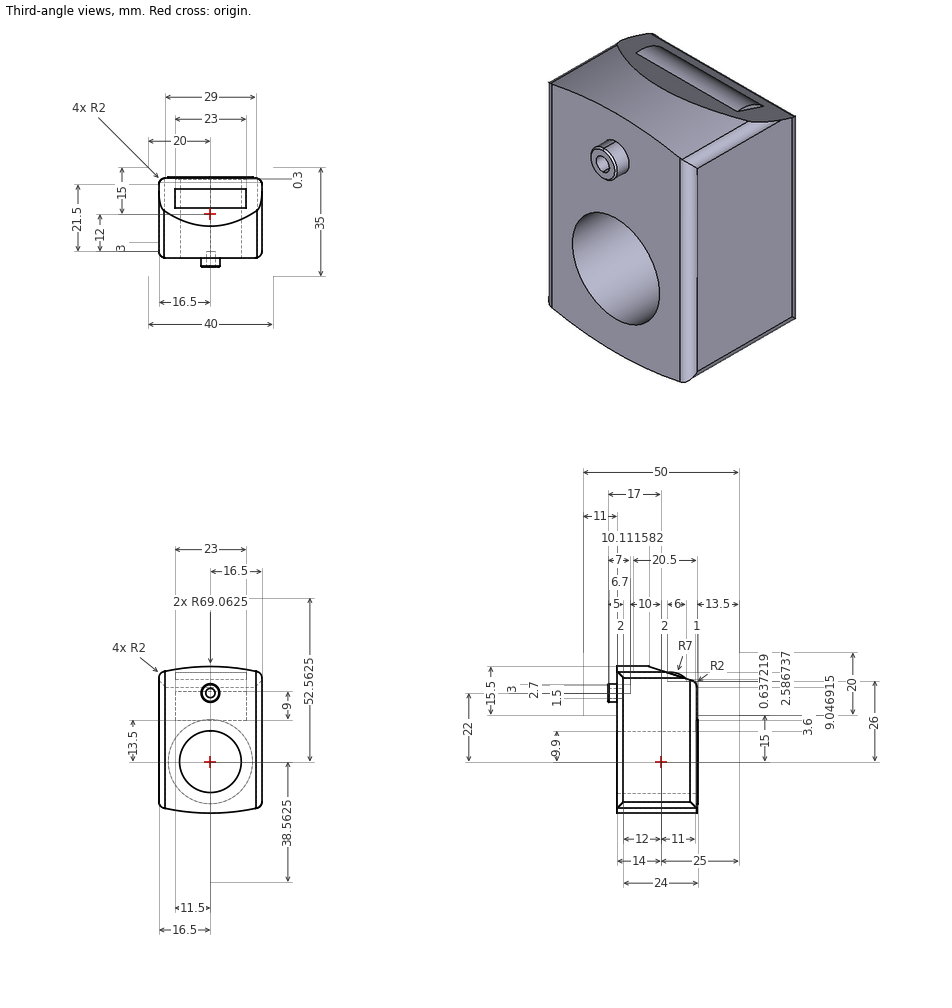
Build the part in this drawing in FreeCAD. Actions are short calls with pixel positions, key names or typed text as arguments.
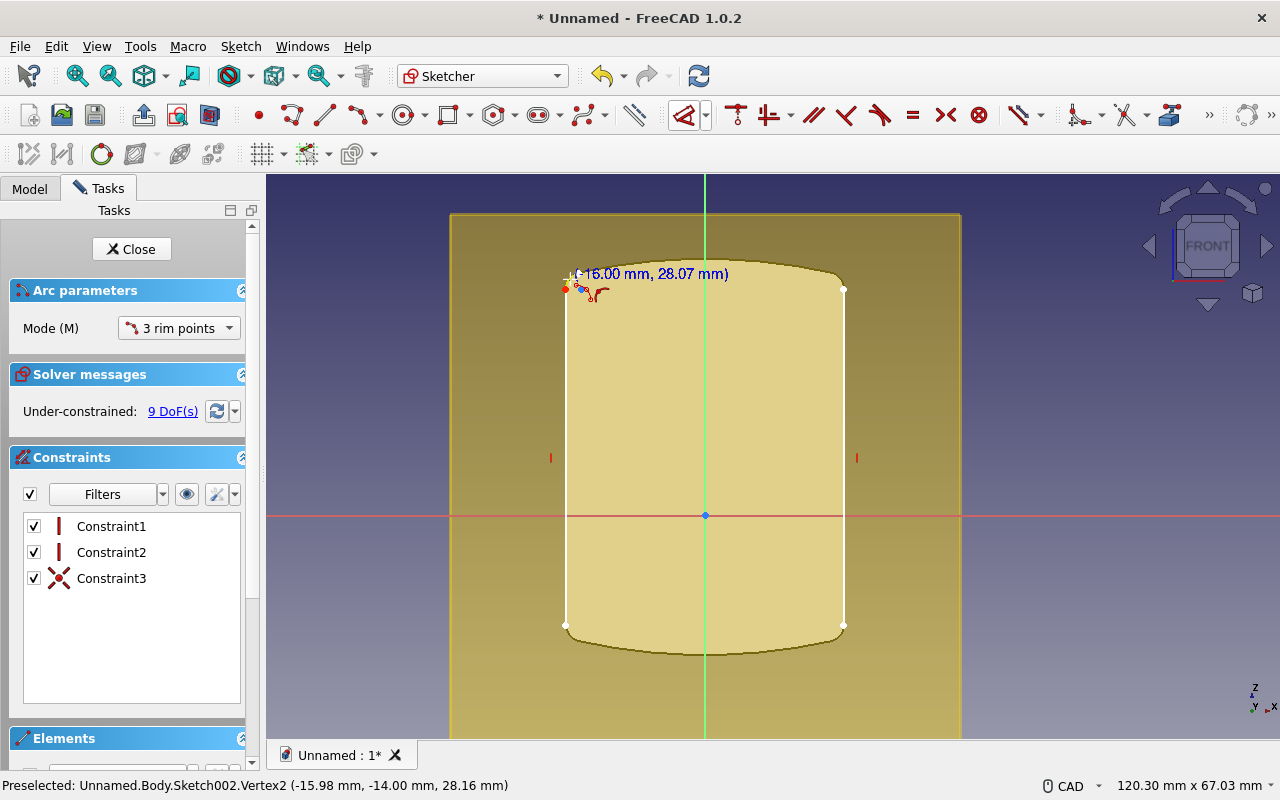
click(579, 274)
click(831, 273)
click(730, 259)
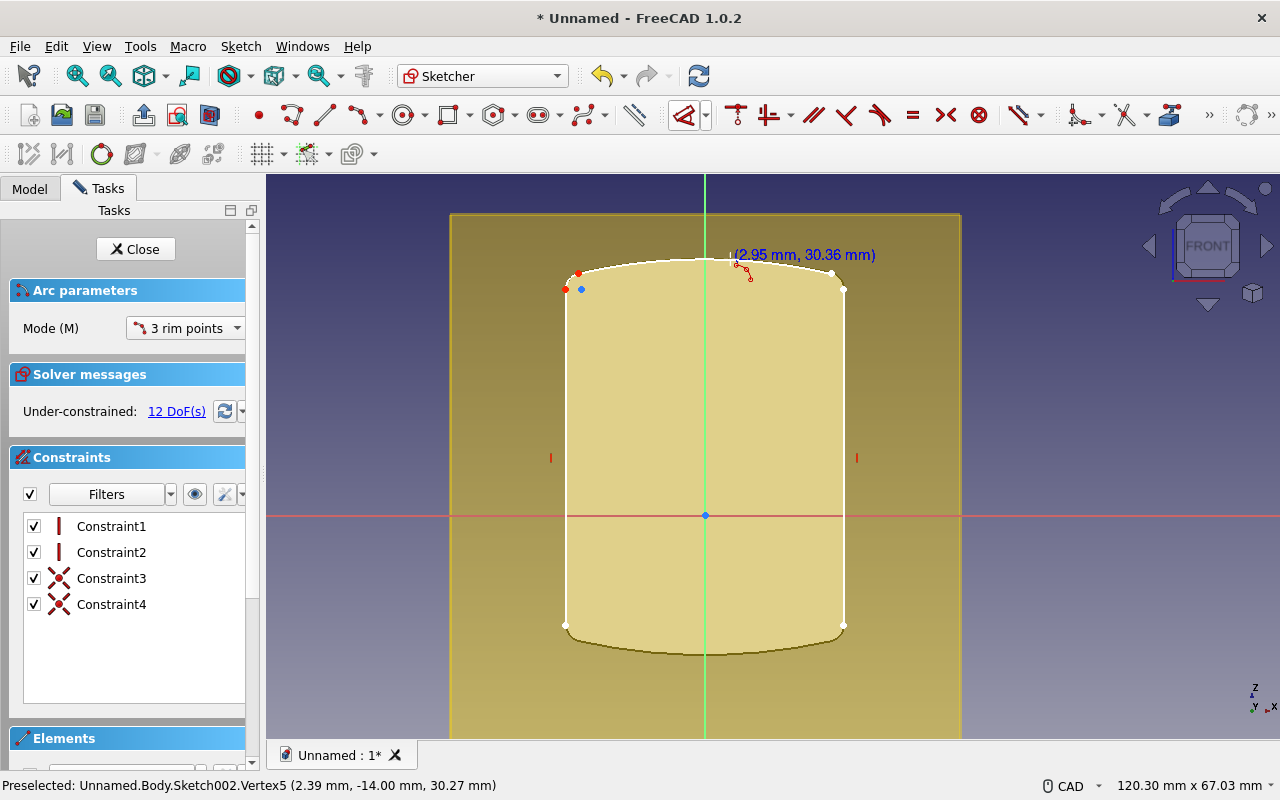
click(831, 274)
click(844, 290)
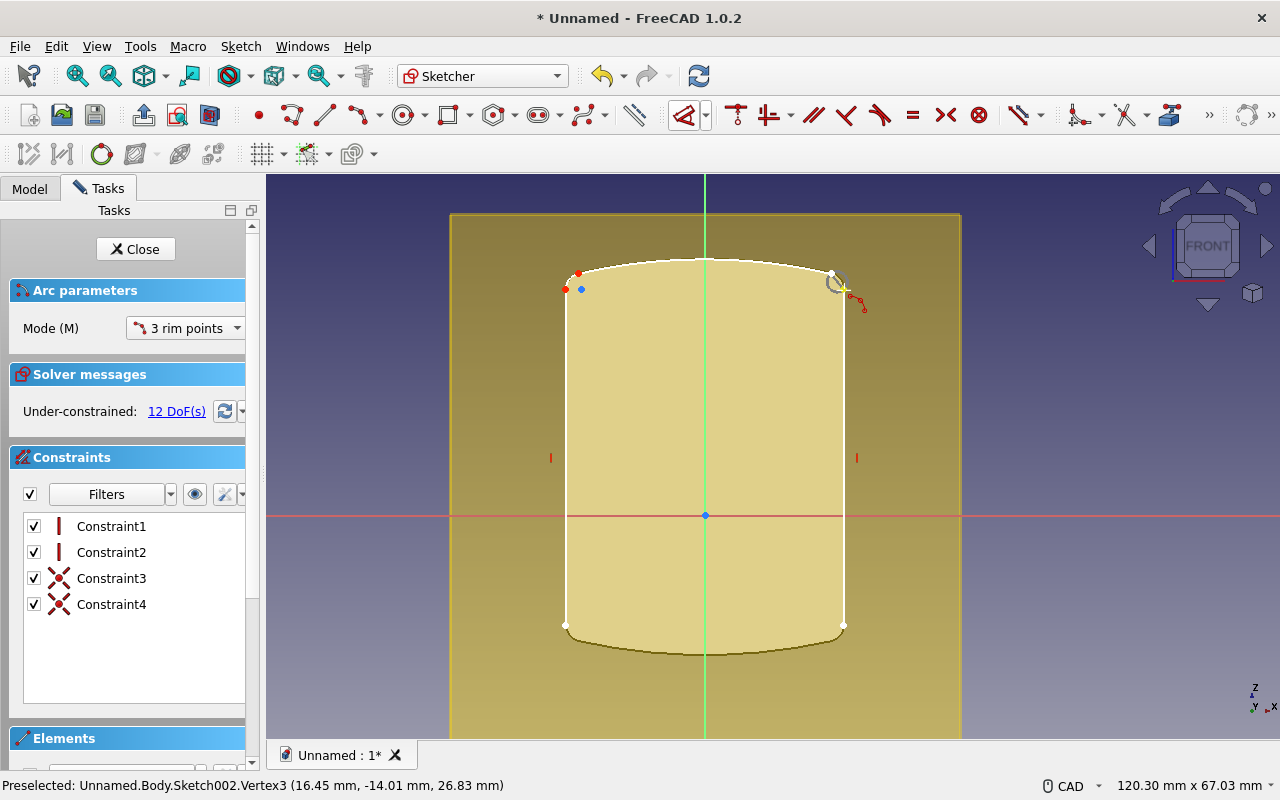
scroll(840, 279, up, 8)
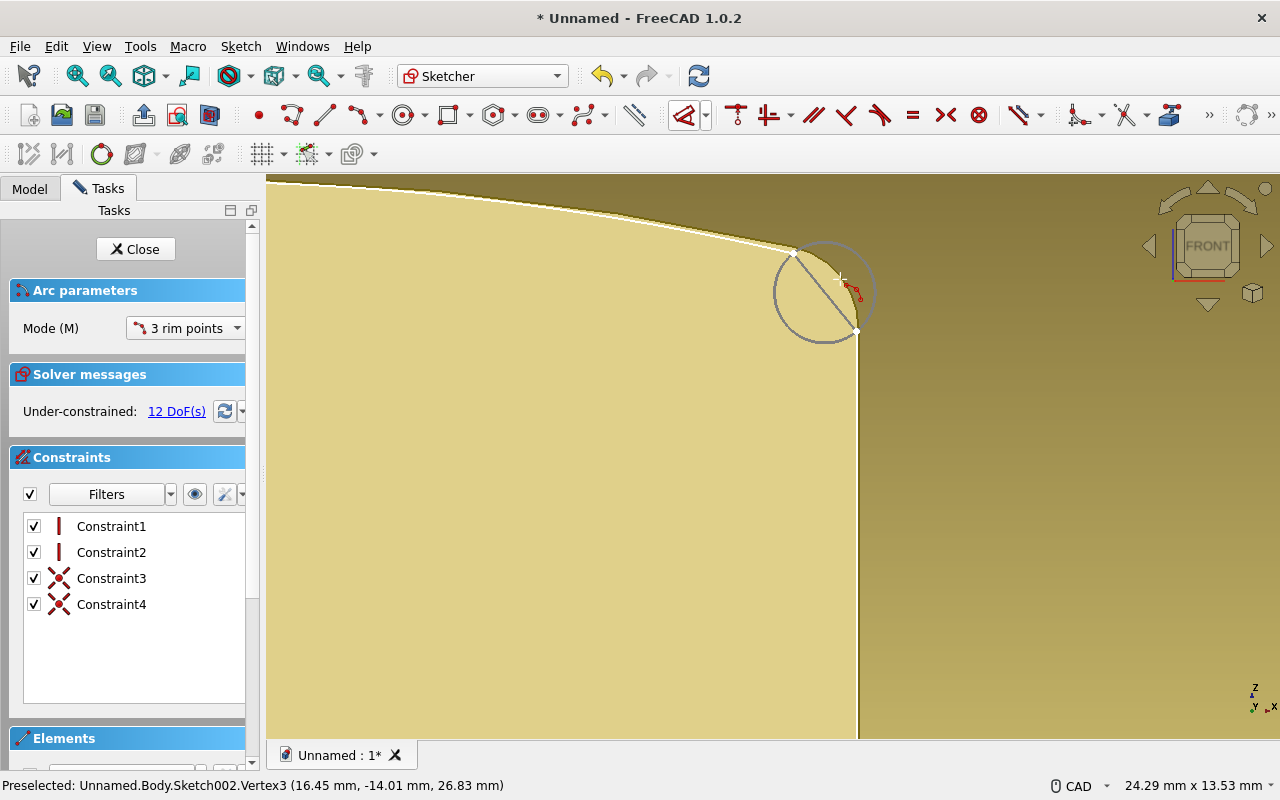
click(840, 276)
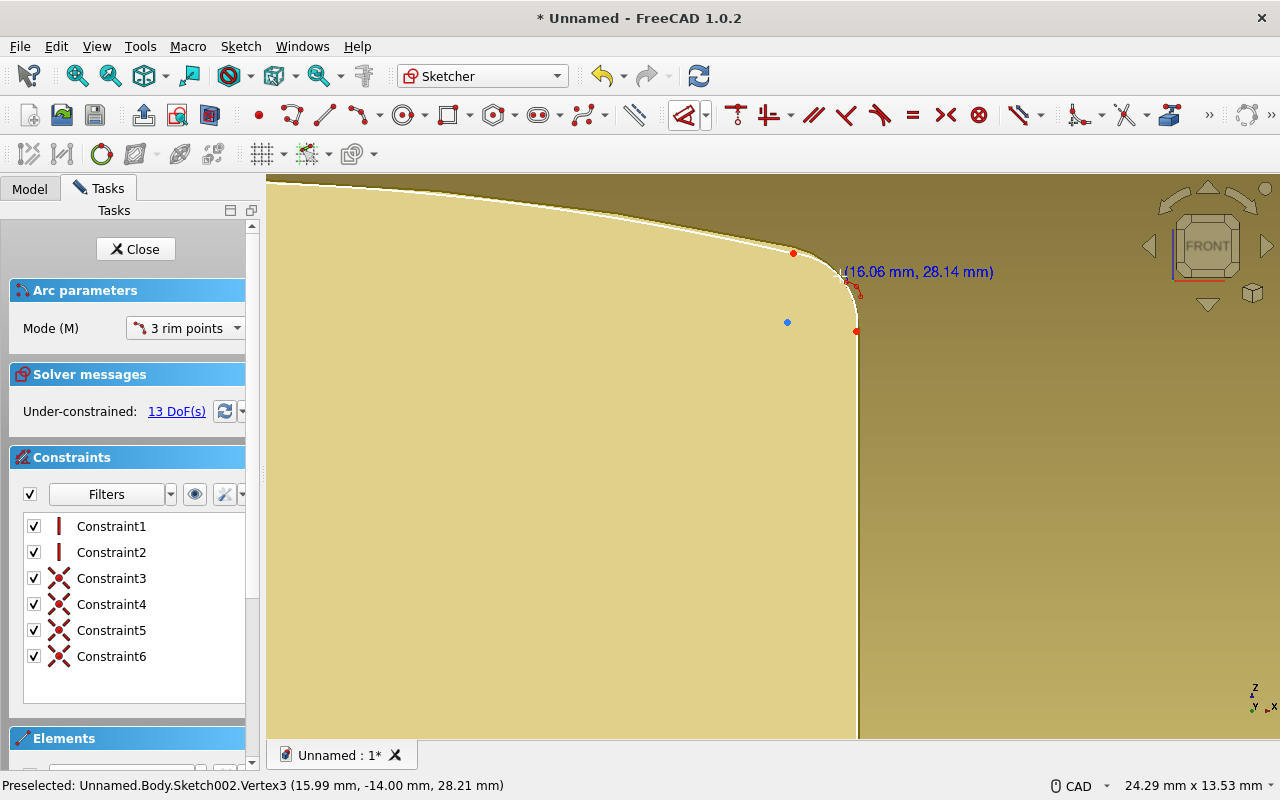
scroll(840, 279, down, 8)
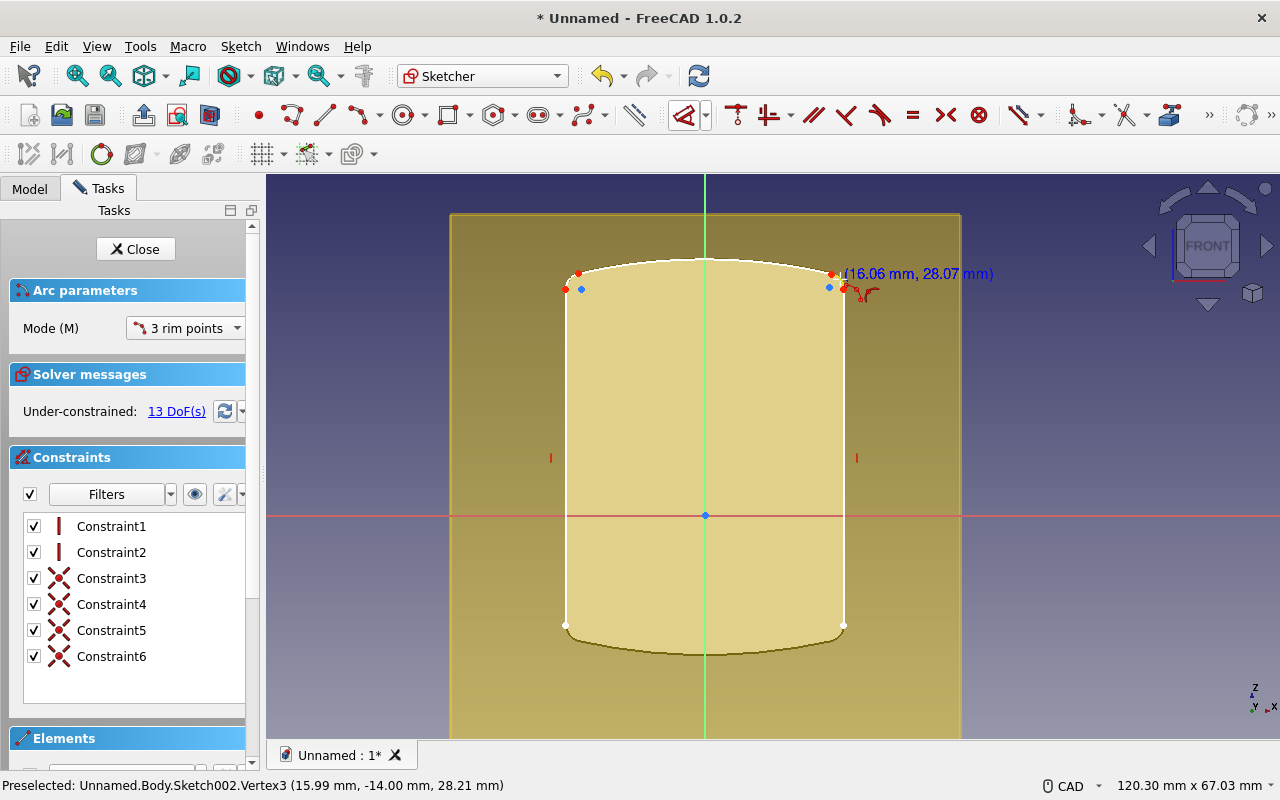
click(844, 626)
click(831, 641)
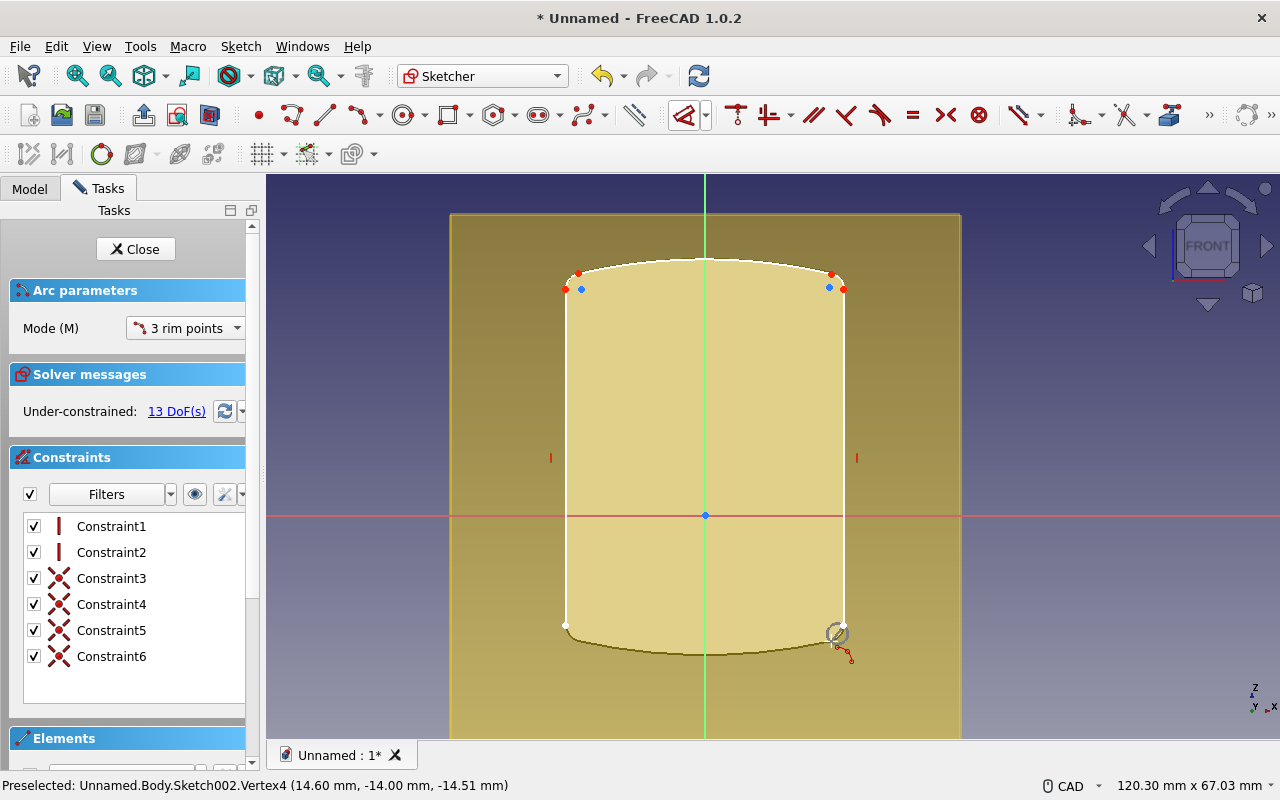
scroll(840, 635, up, 8)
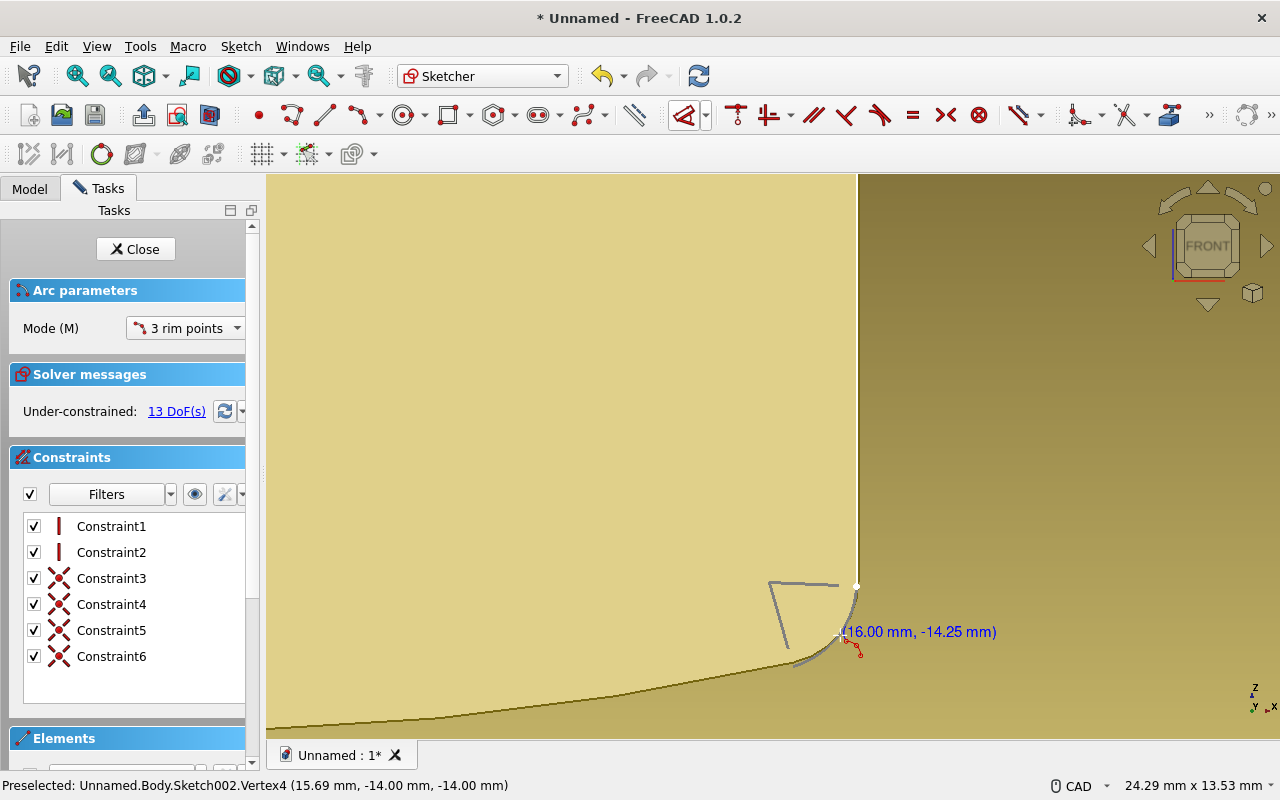
click(840, 633)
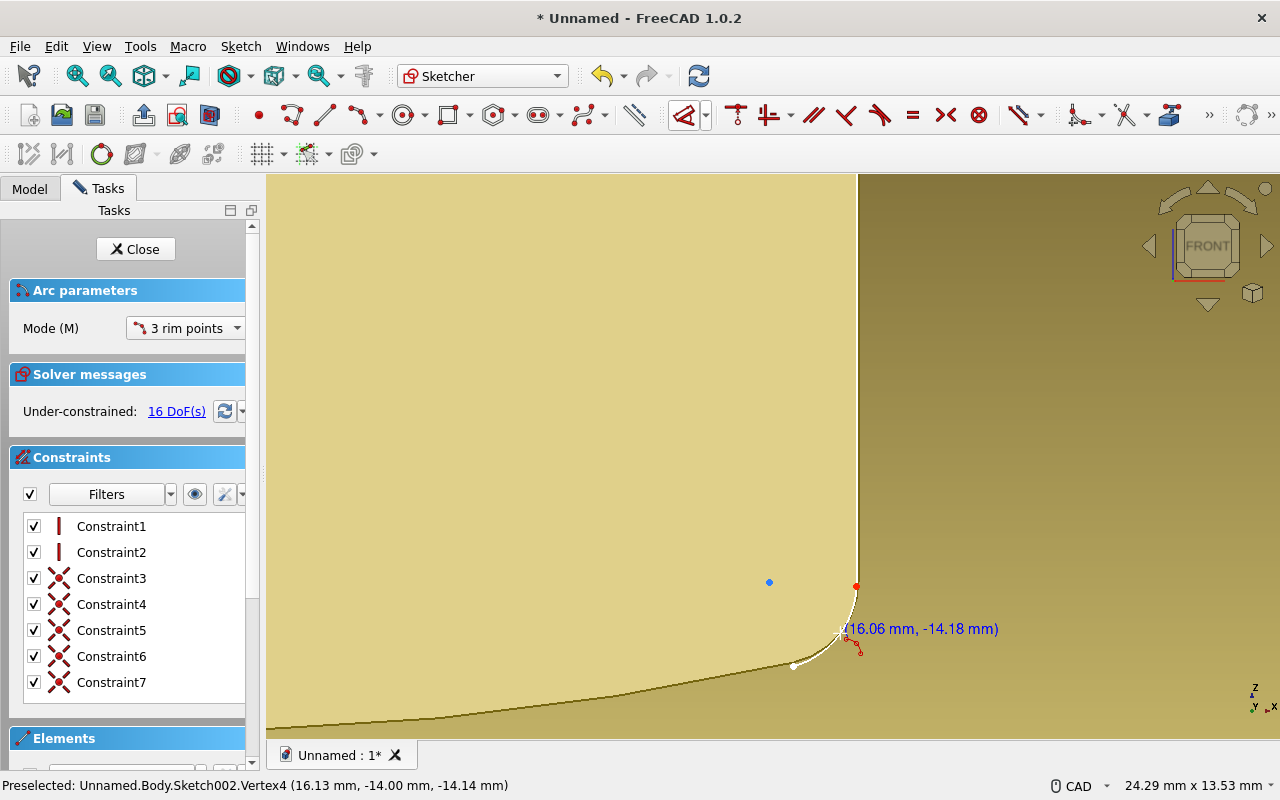
scroll(840, 635, down, 8)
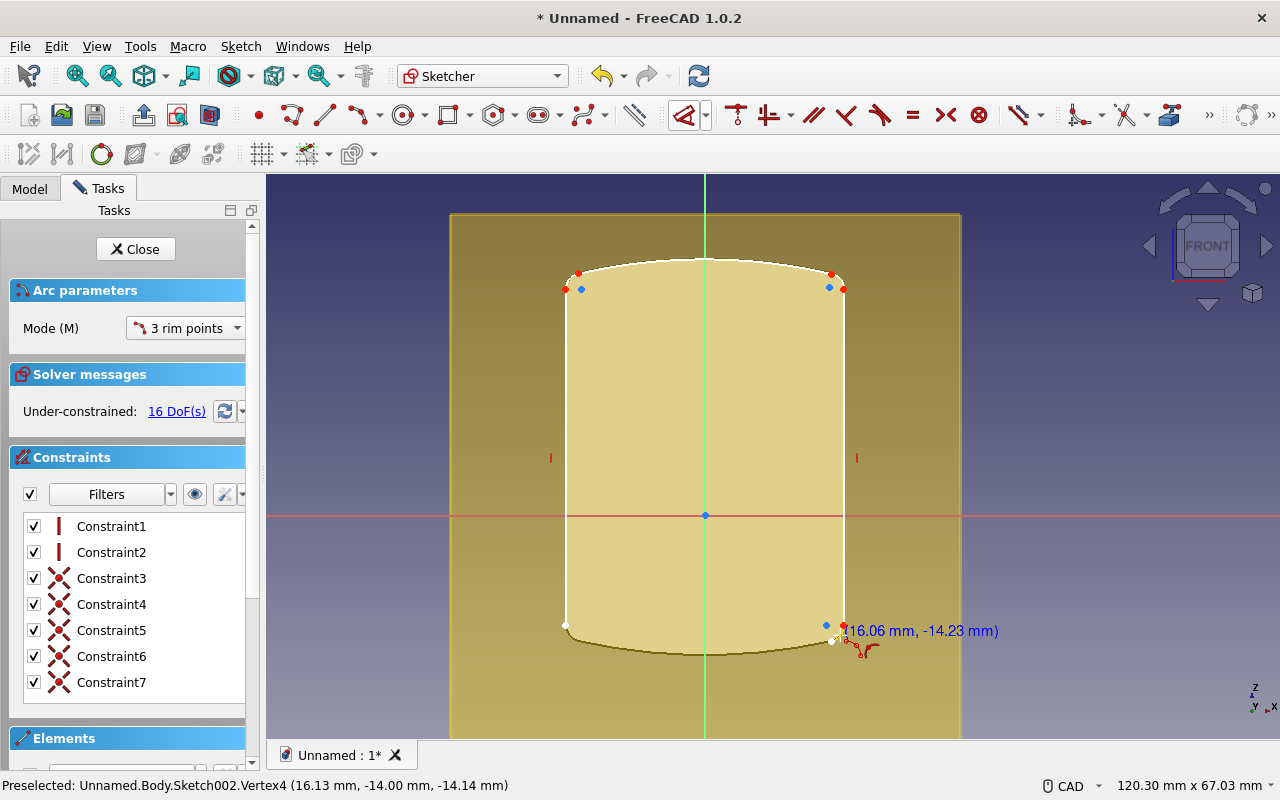
click(831, 642)
click(579, 641)
click(680, 654)